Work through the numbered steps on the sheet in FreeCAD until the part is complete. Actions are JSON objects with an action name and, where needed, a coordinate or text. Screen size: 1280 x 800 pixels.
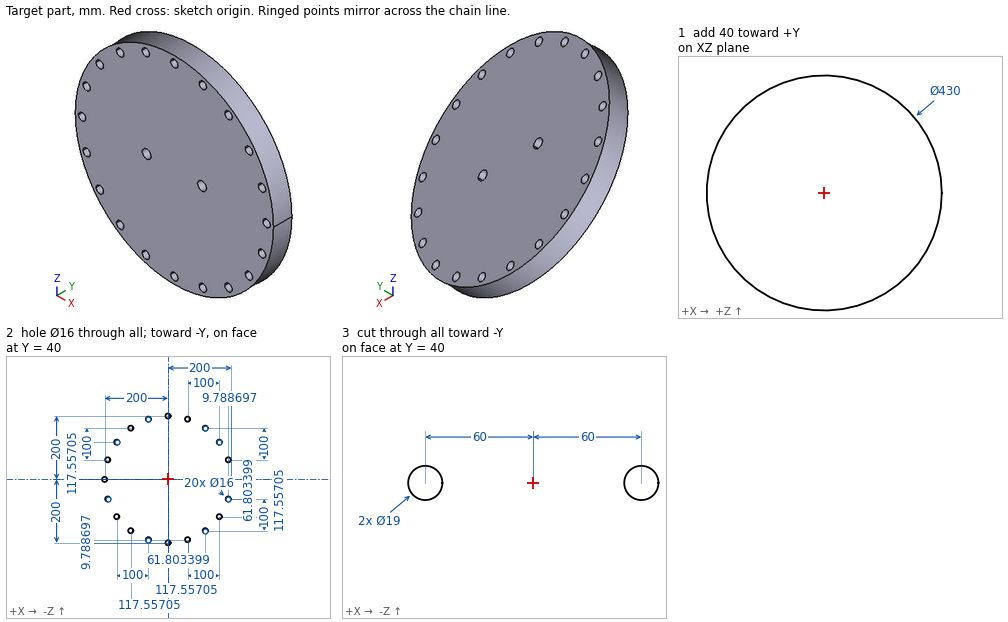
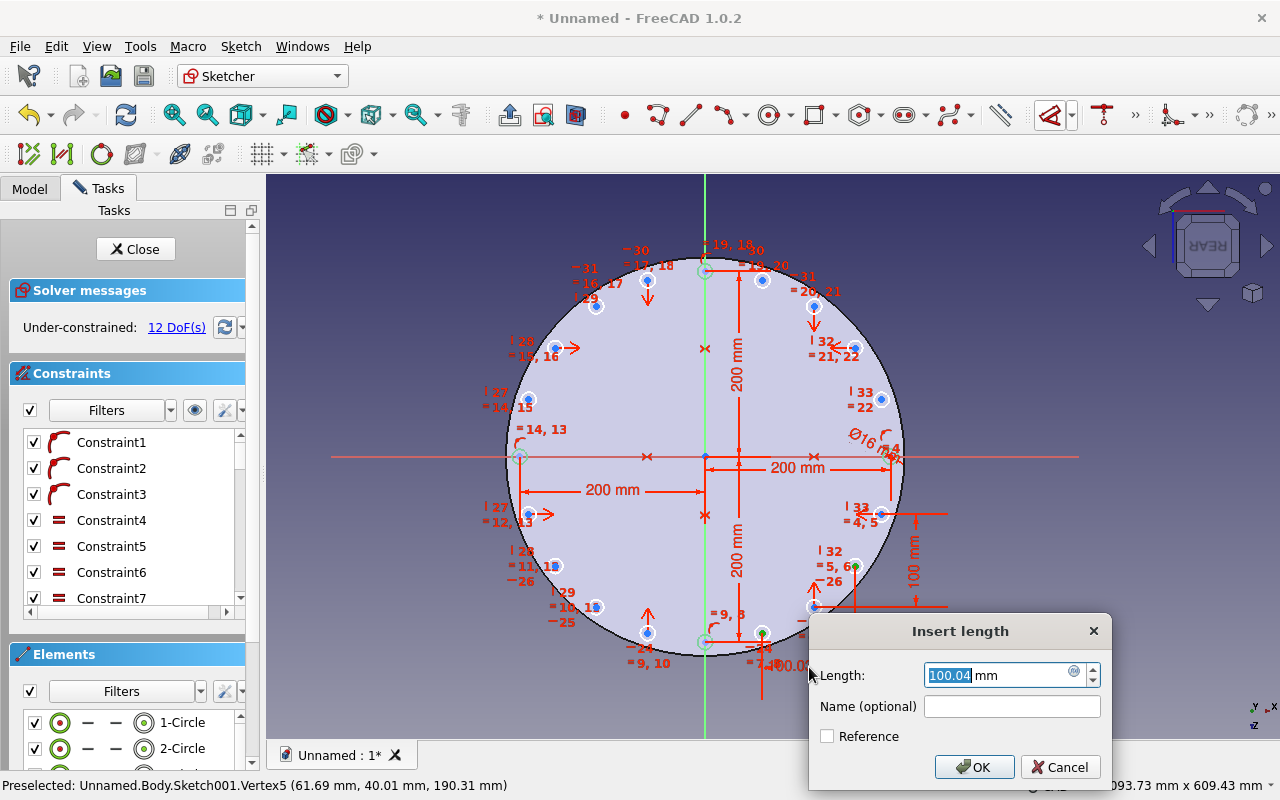
{"action": "type", "text": "100"}
{"action": "key", "text": "Return"}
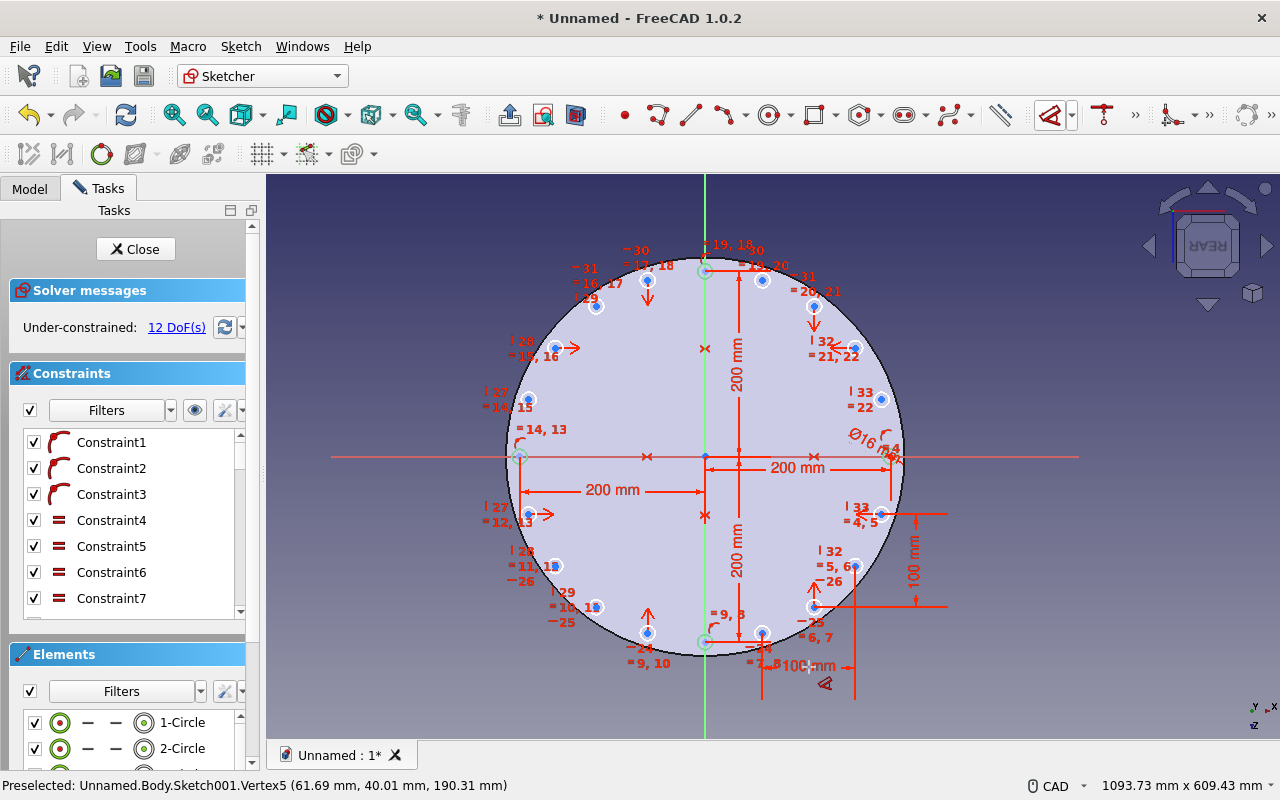
{"action": "left_click", "coordinate": [648, 633]}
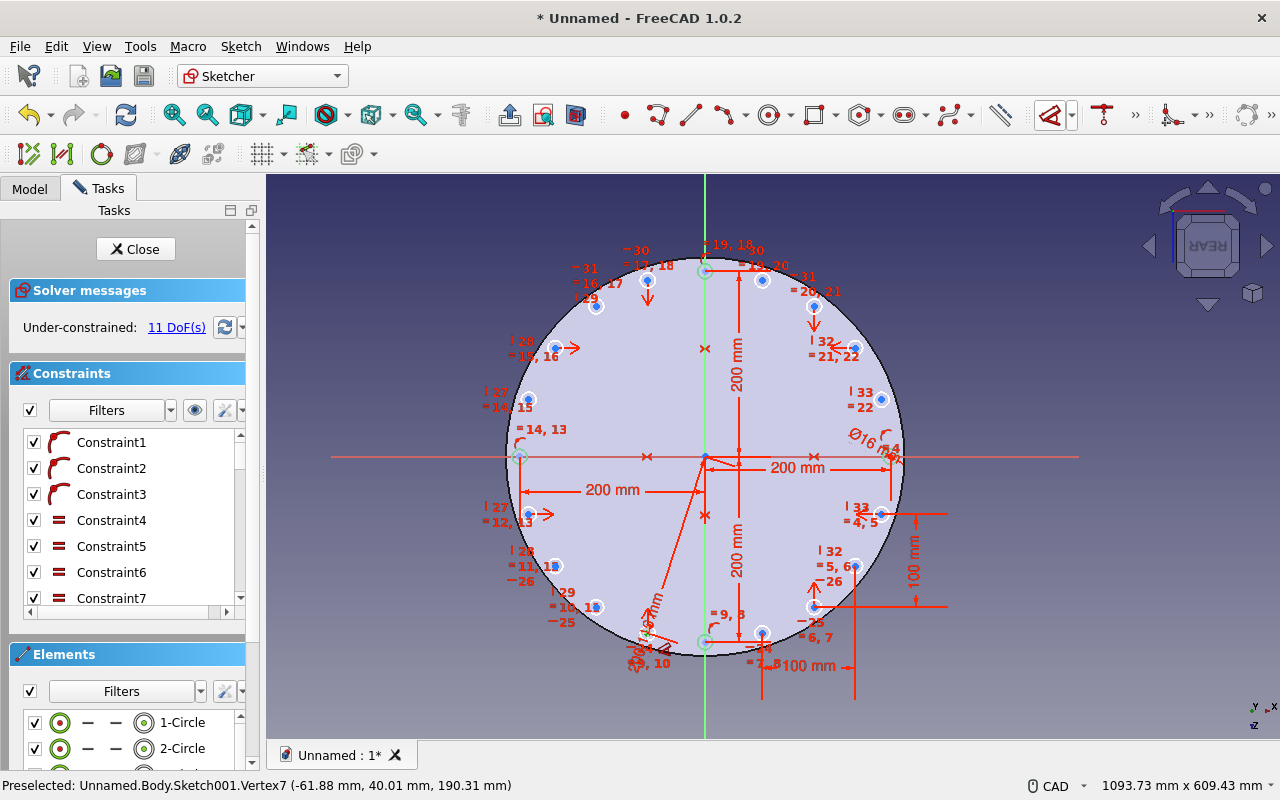
{"action": "left_click", "coordinate": [555, 566]}
{"action": "left_click", "coordinate": [602, 667]}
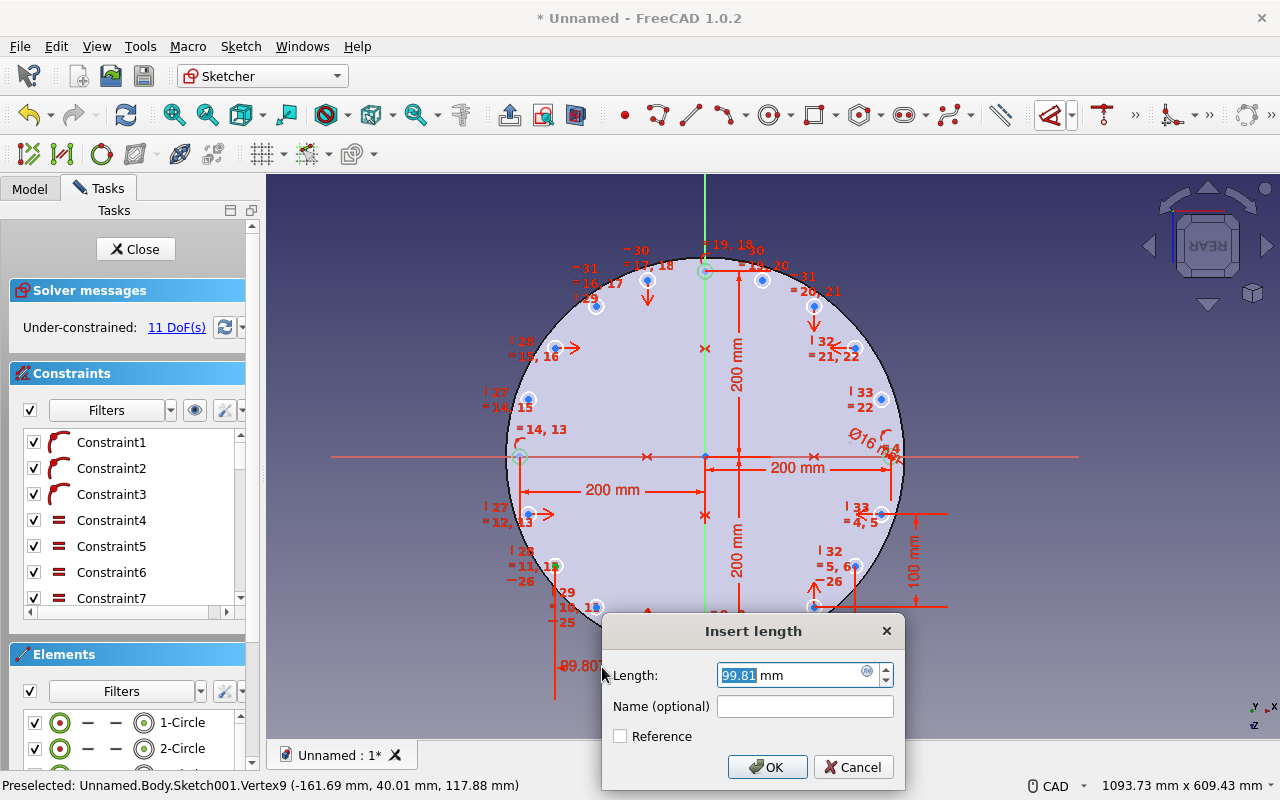
{"action": "type", "text": "100"}
{"action": "key", "text": "Return"}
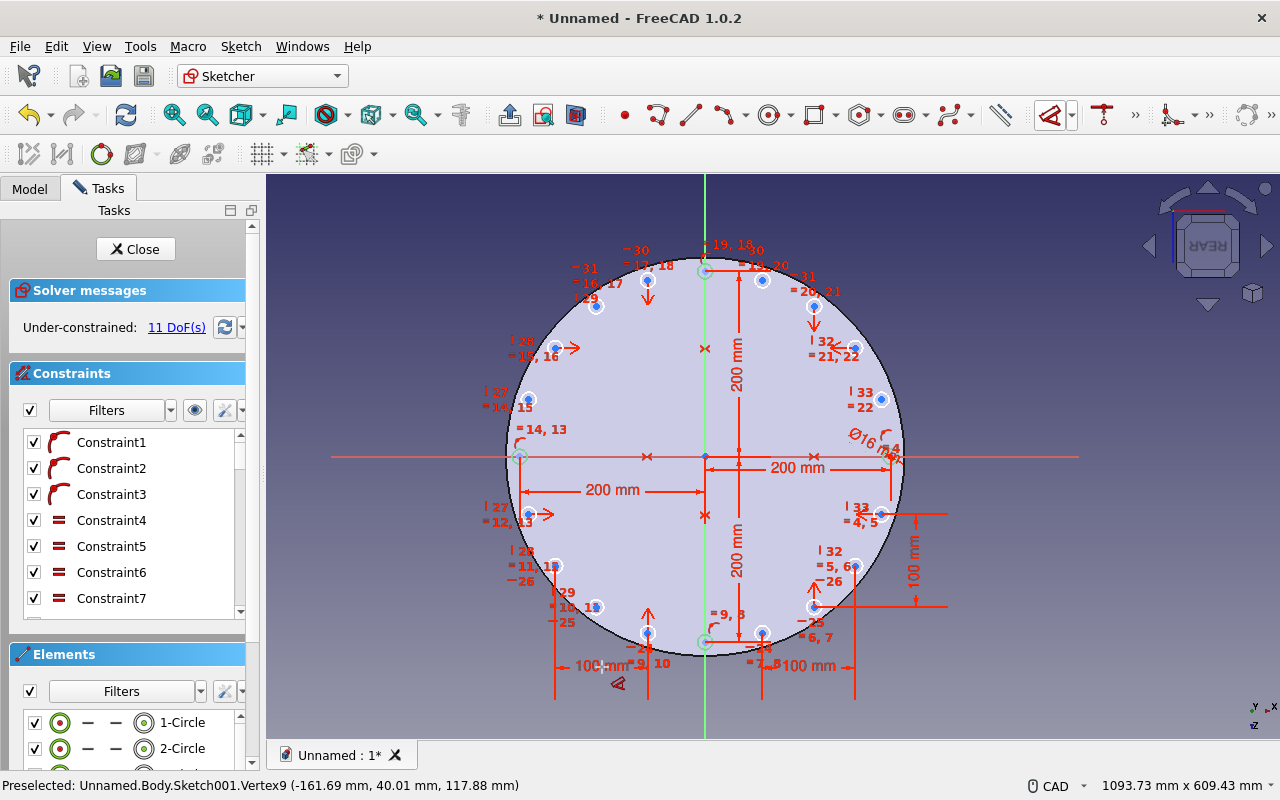
{"action": "left_click", "coordinate": [529, 400]}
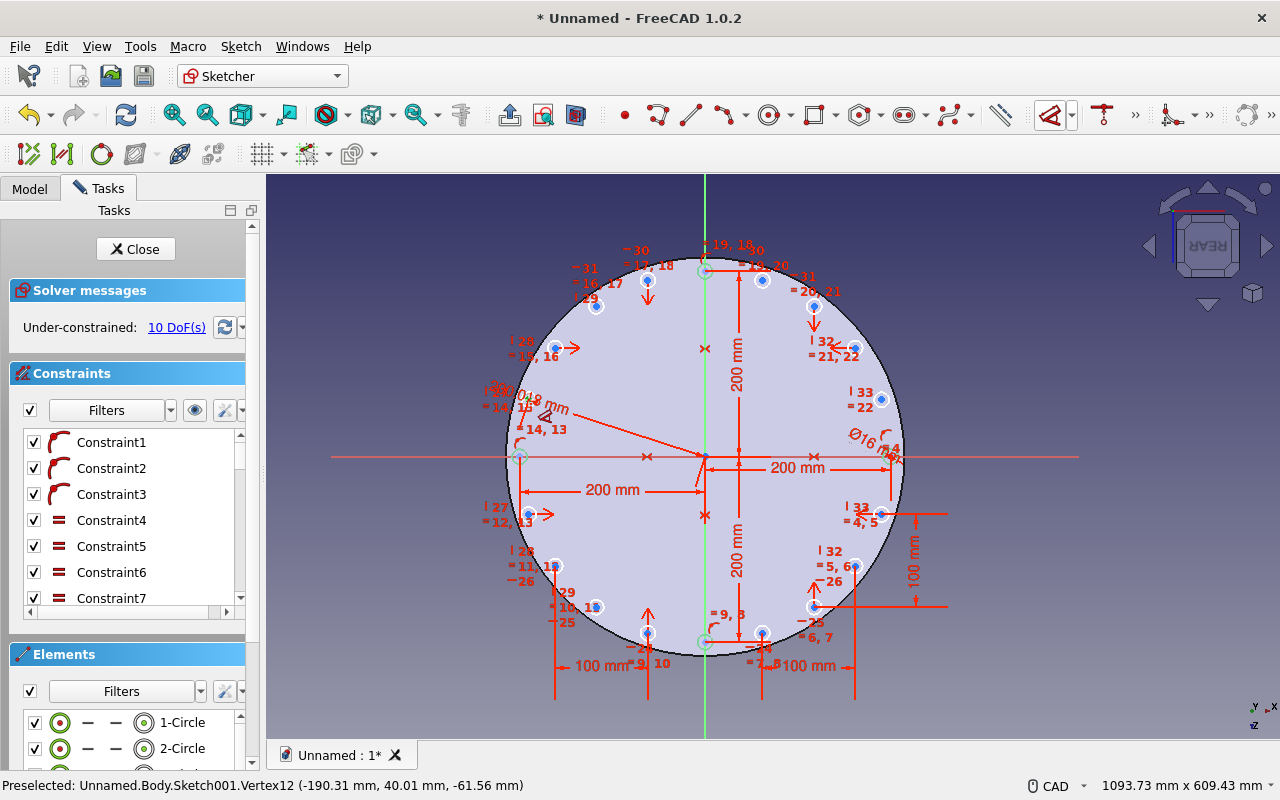
{"action": "left_click", "coordinate": [596, 306]}
{"action": "left_click", "coordinate": [495, 353]}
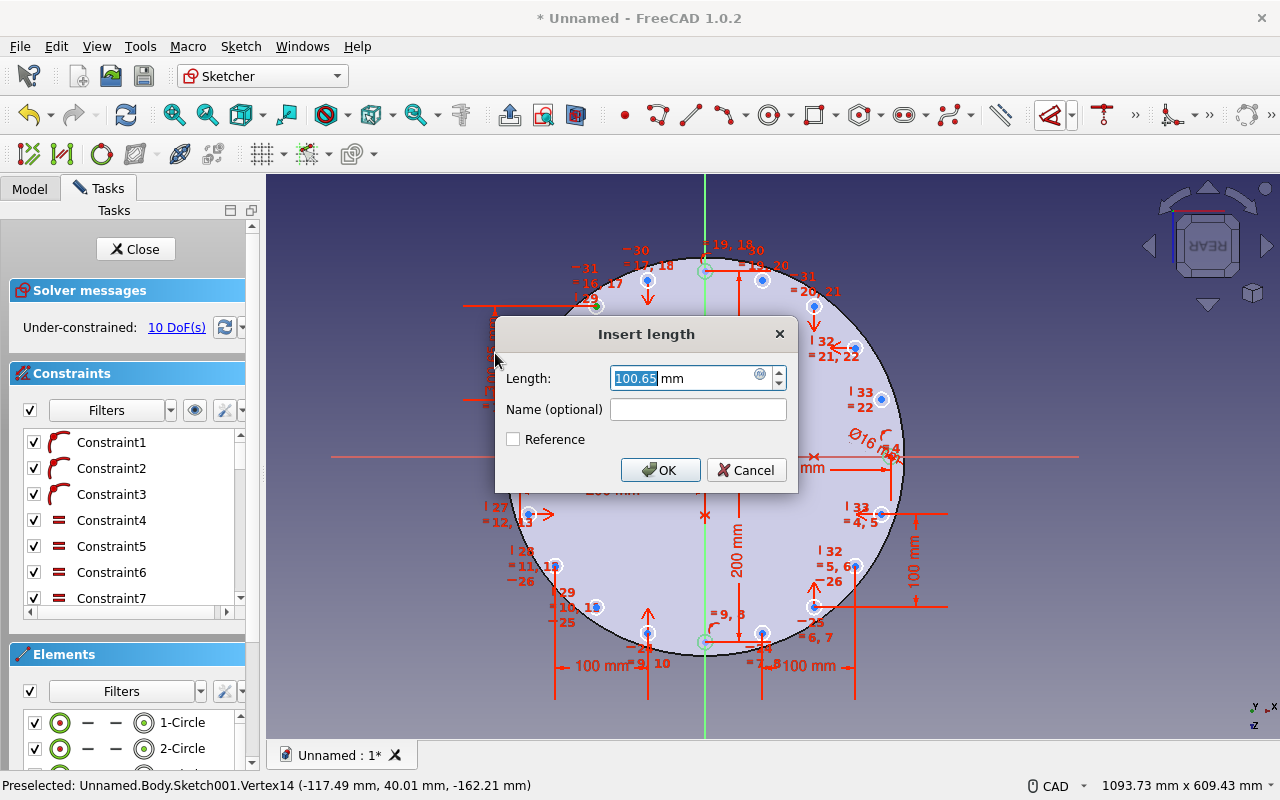
{"action": "type", "text": "100"}
{"action": "key", "text": "Return"}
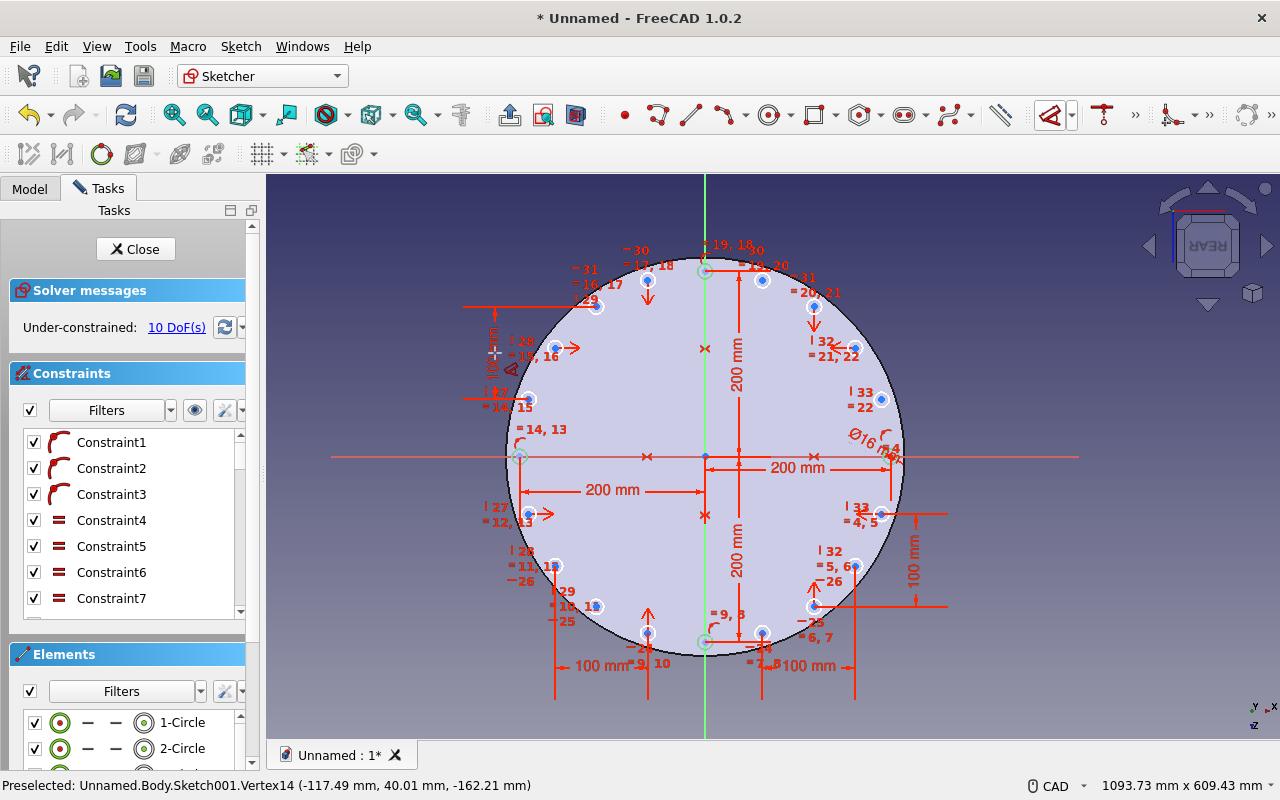
{"action": "left_click", "coordinate": [763, 280]}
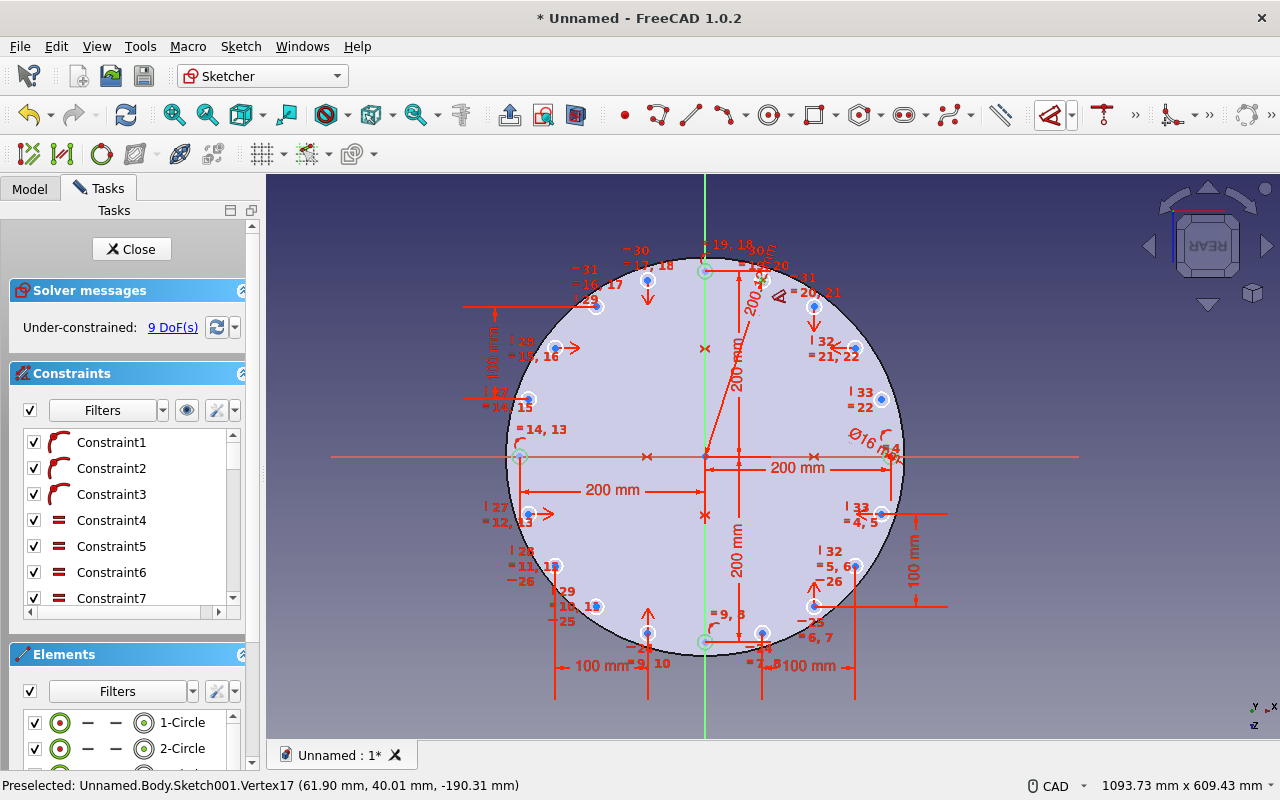
{"action": "left_click", "coordinate": [855, 348]}
{"action": "left_click", "coordinate": [809, 246]}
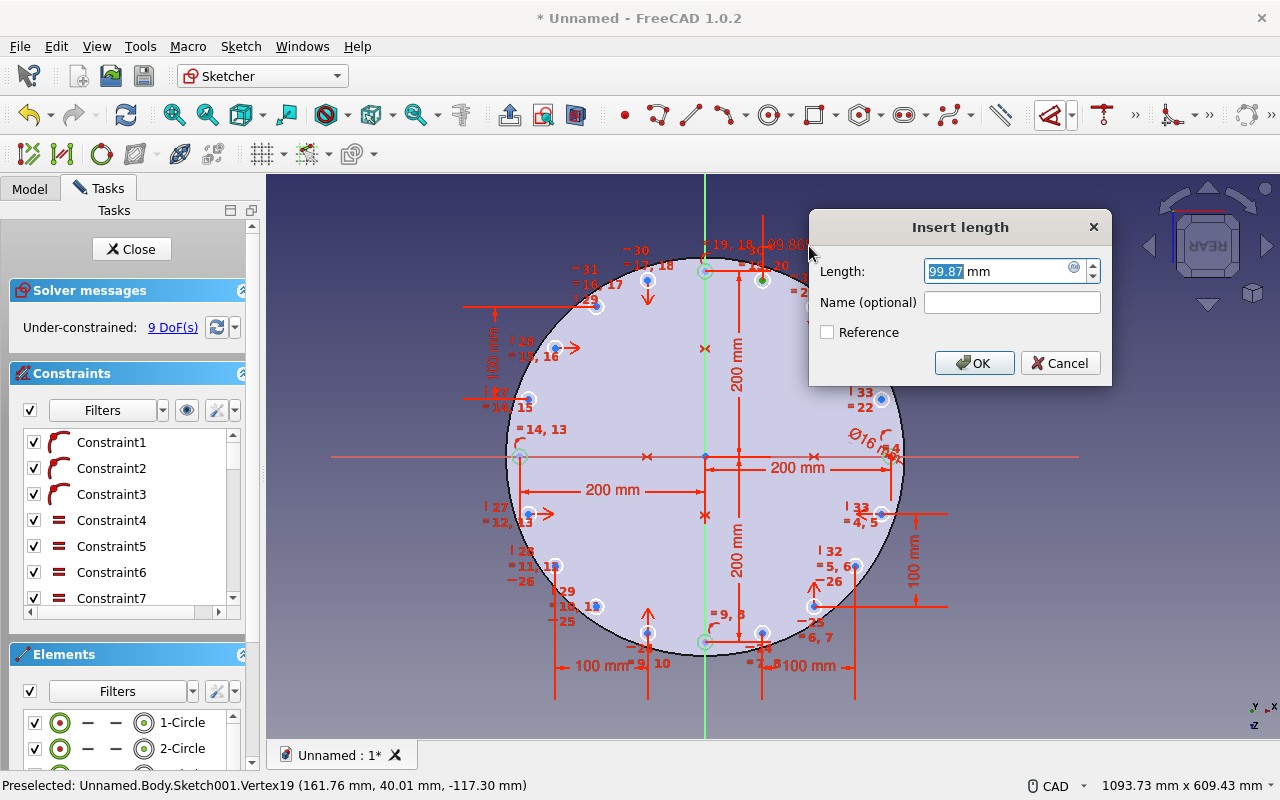
{"action": "type", "text": "100"}
{"action": "key", "text": "Return"}